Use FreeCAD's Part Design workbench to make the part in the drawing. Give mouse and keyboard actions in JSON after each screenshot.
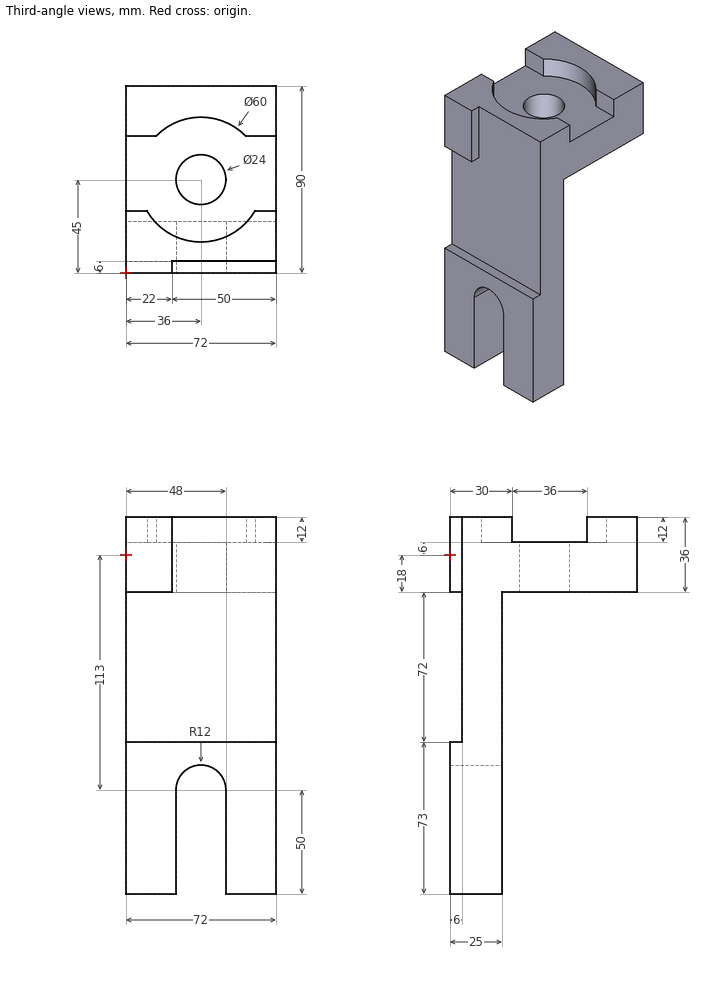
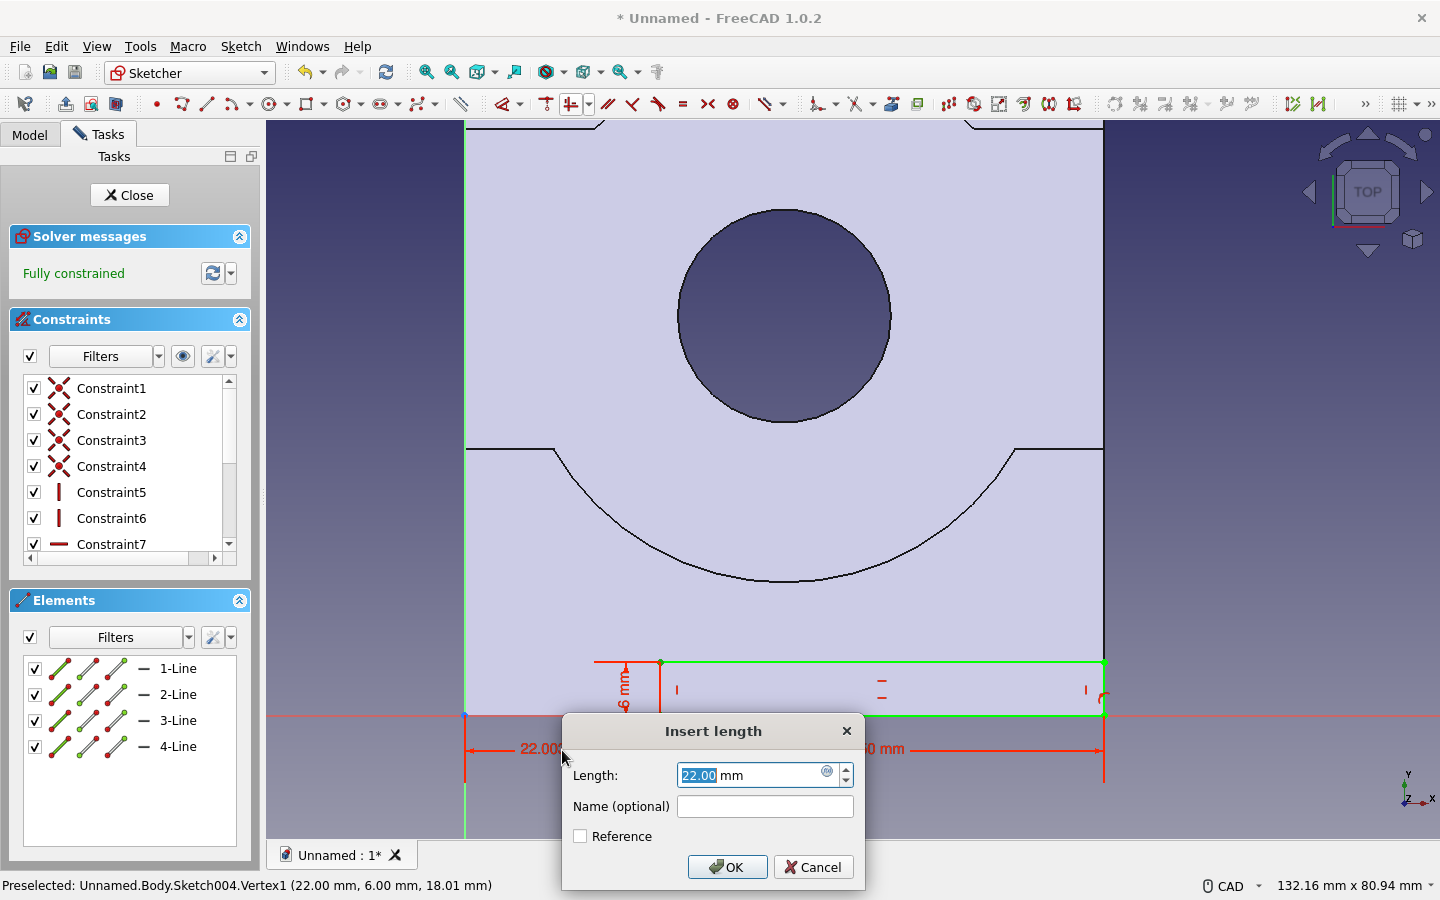
{"action": "type", "text": "22"}
{"action": "key", "text": "Return"}
{"action": "key", "text": "Escape"}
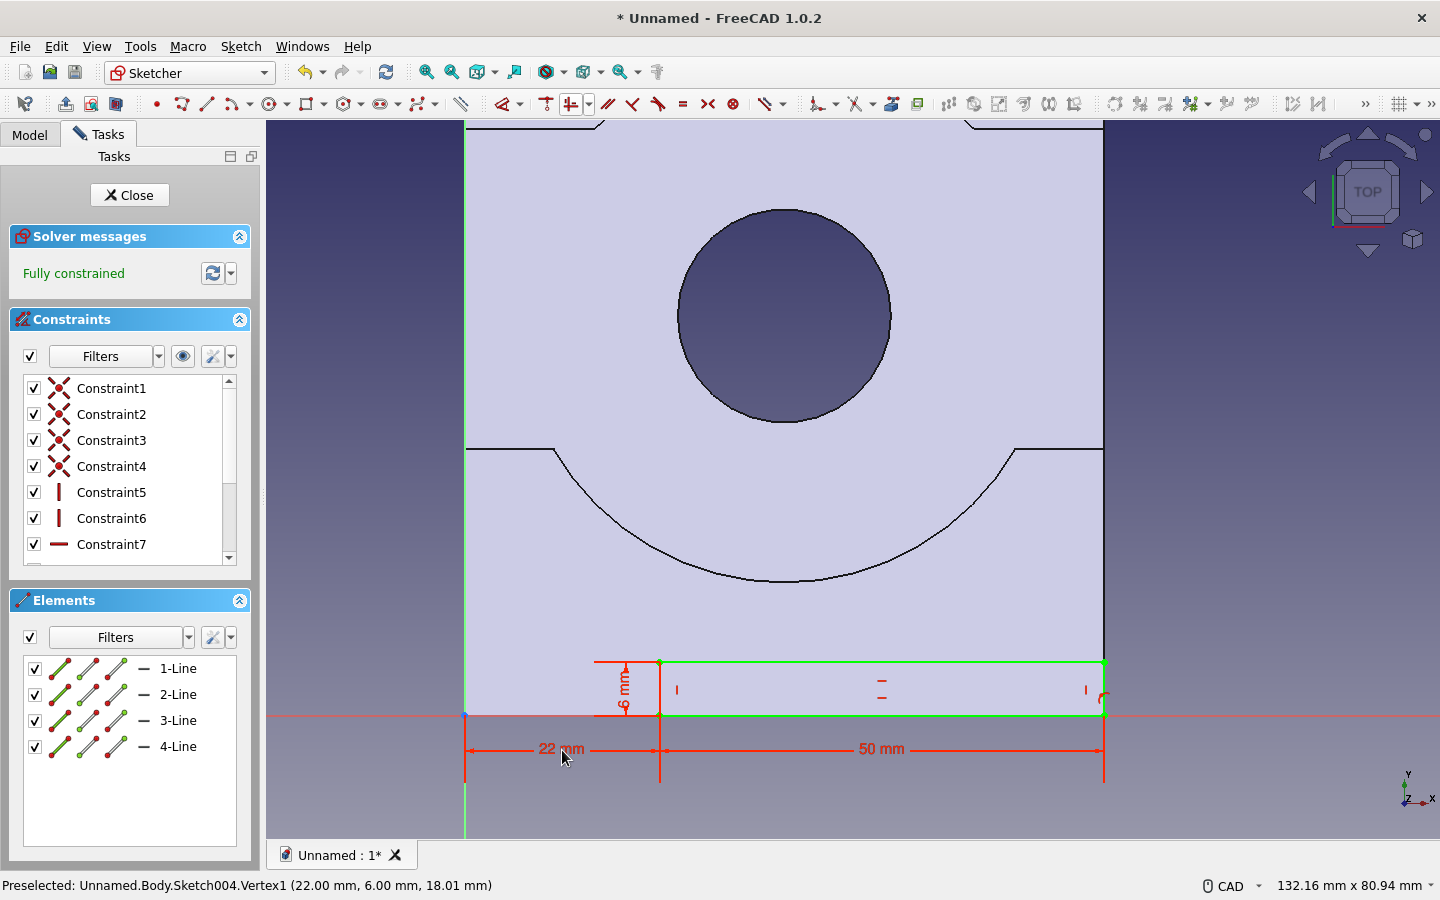
{"action": "left_click", "coordinate": [130, 195]}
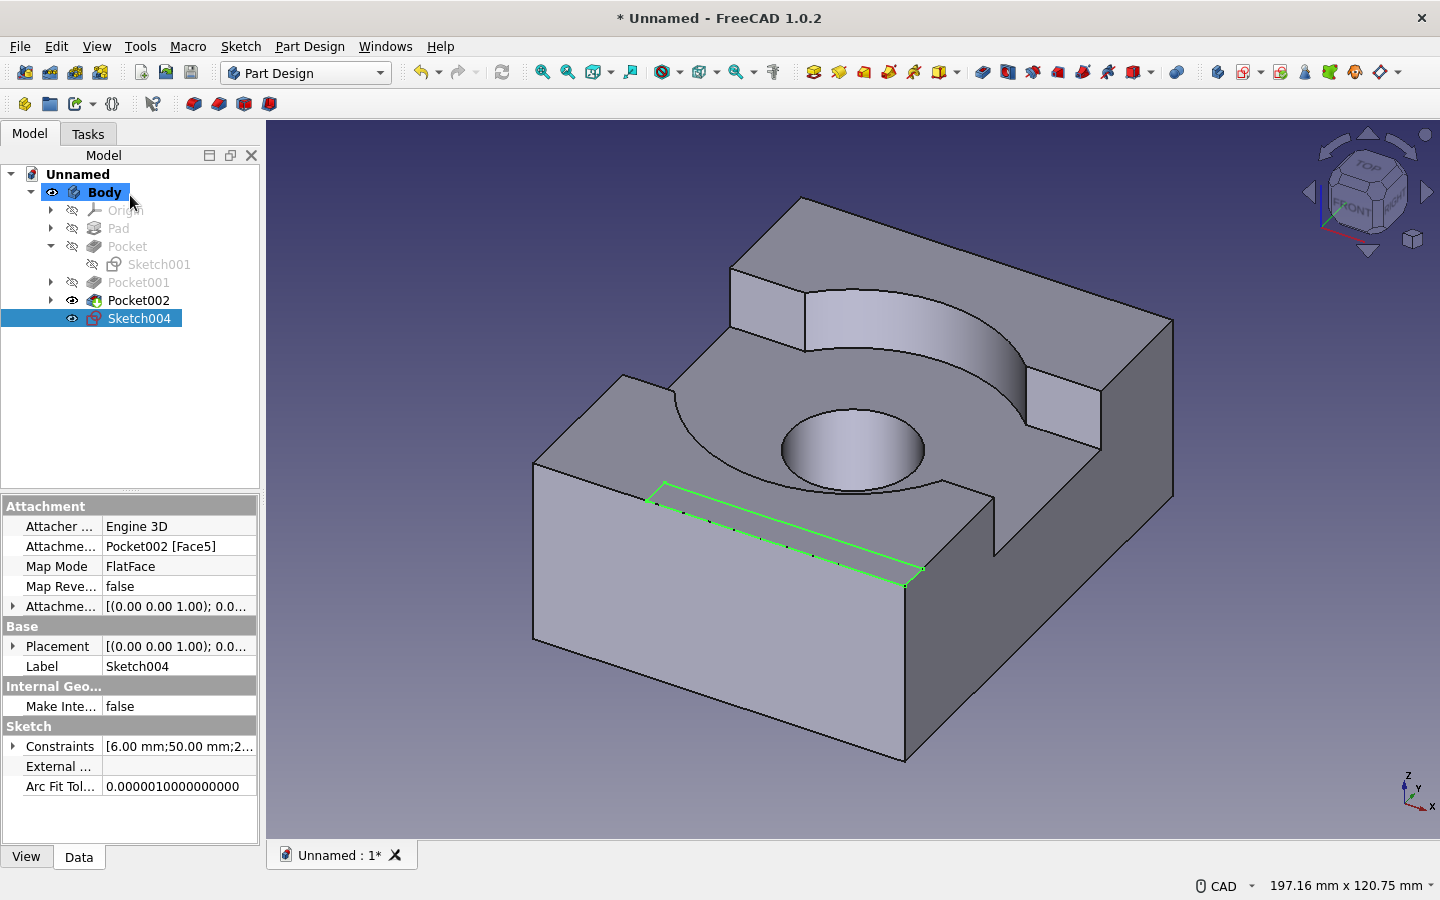
{"action": "left_click", "coordinate": [983, 72]}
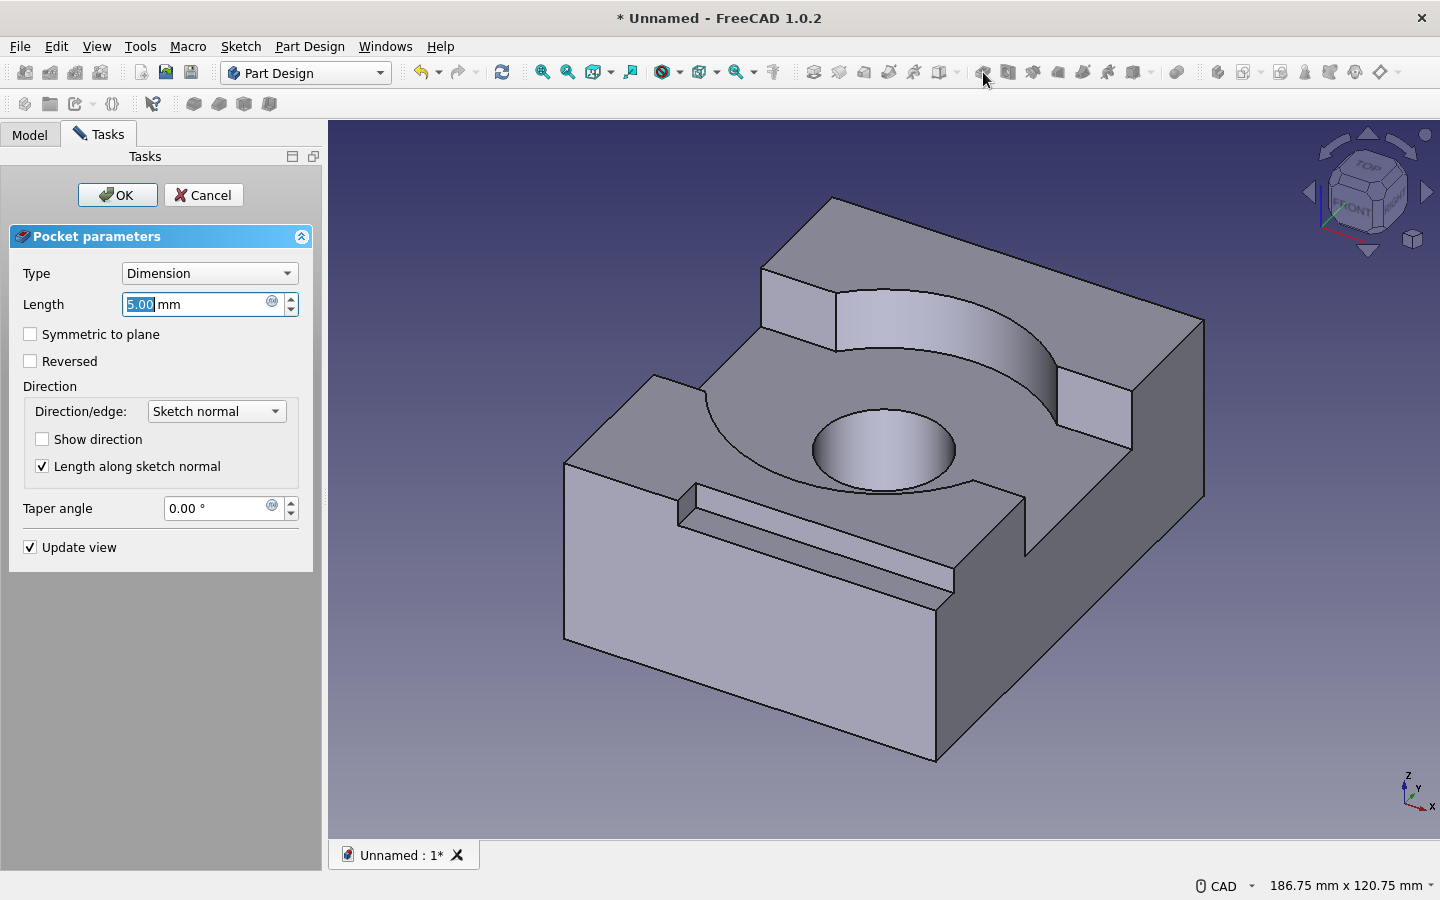
{"action": "left_click", "coordinate": [210, 274]}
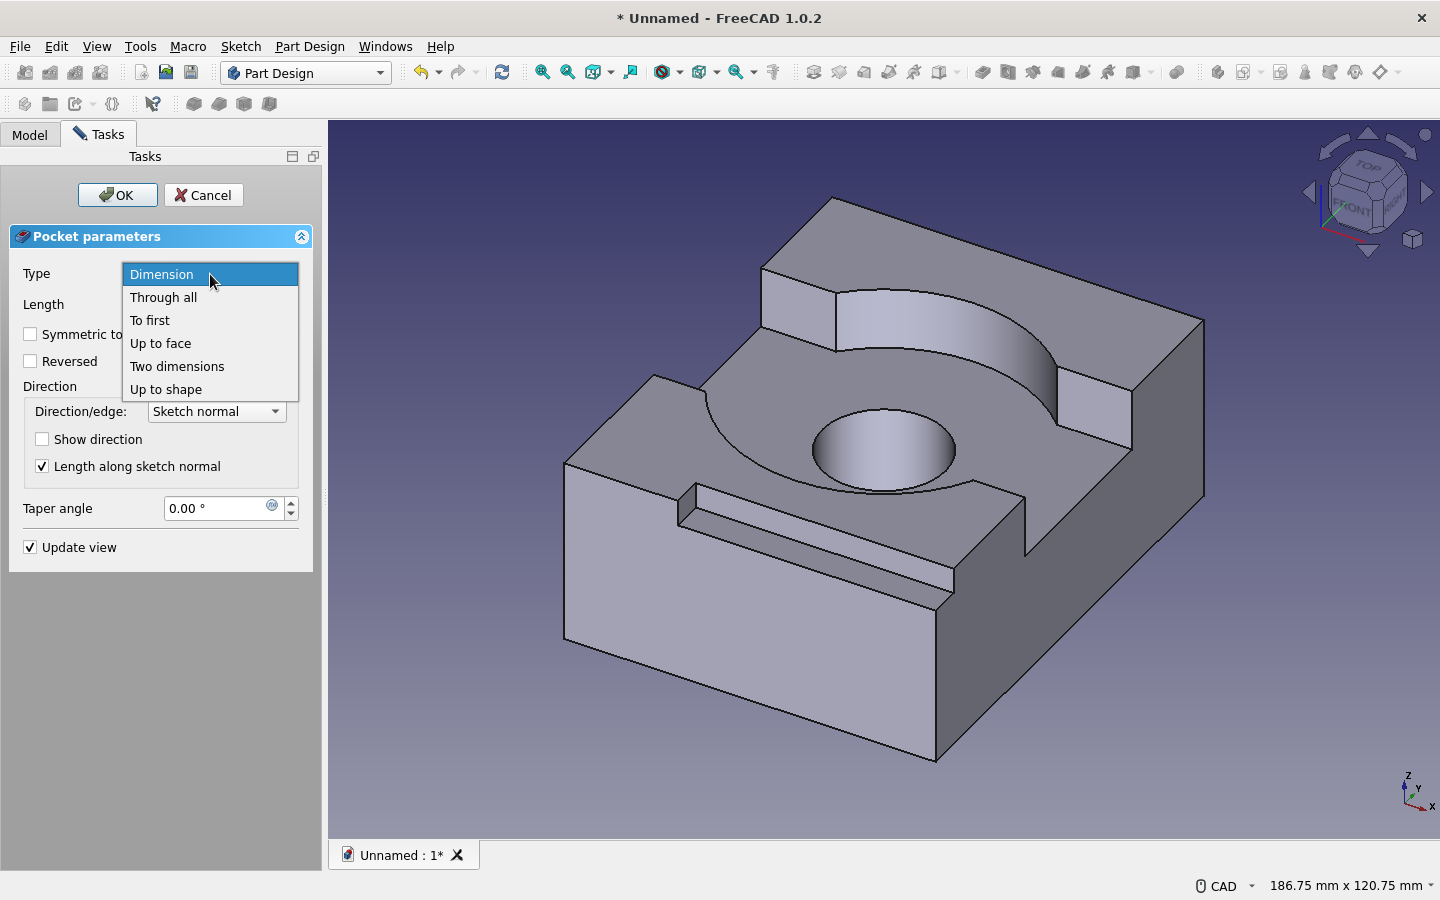
{"action": "left_click", "coordinate": [208, 298]}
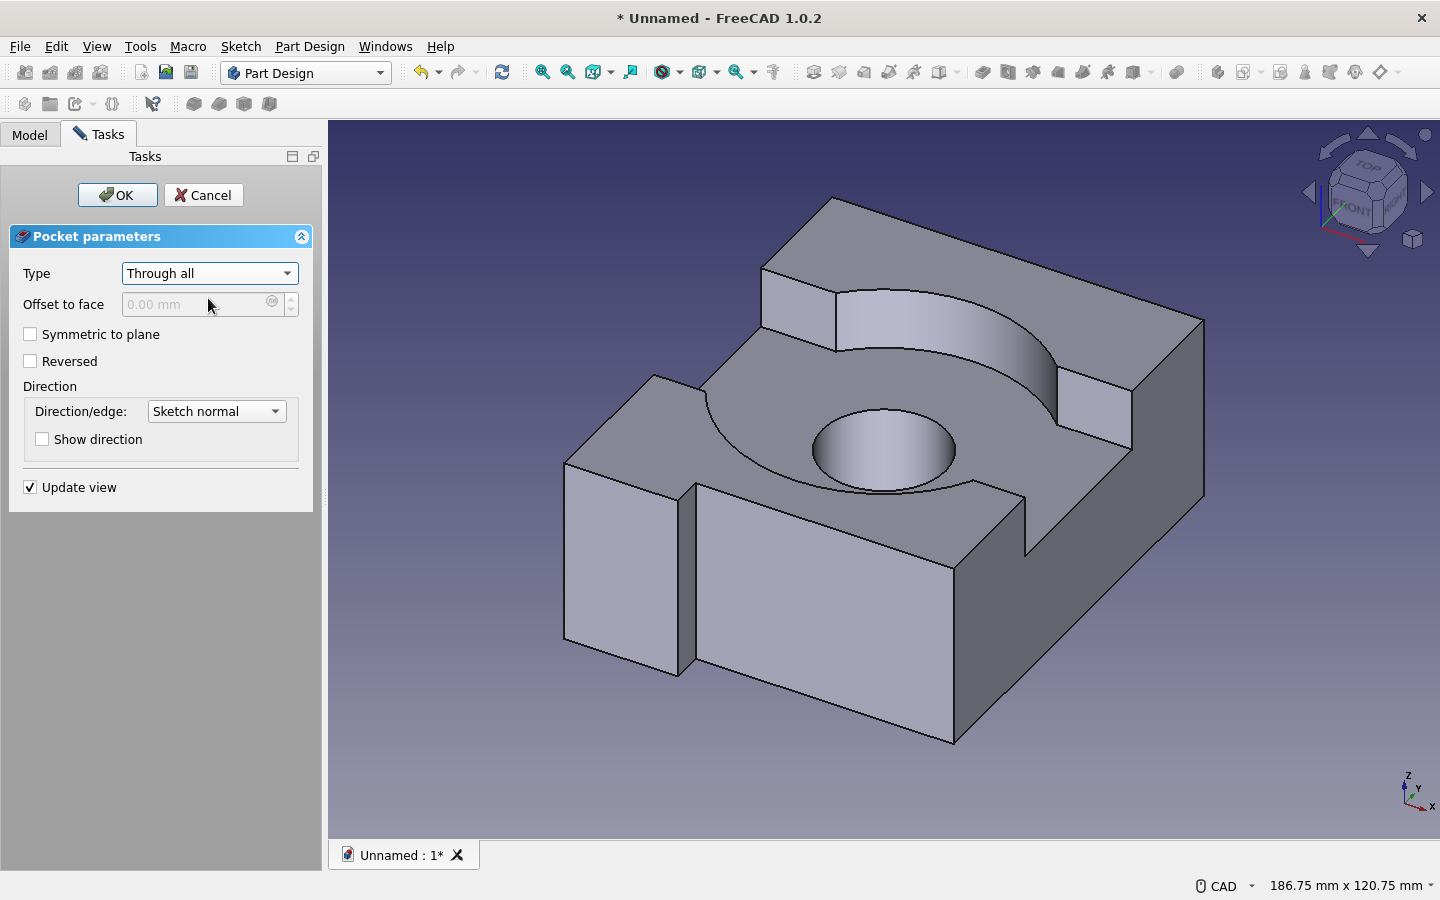
{"action": "left_click", "coordinate": [118, 195]}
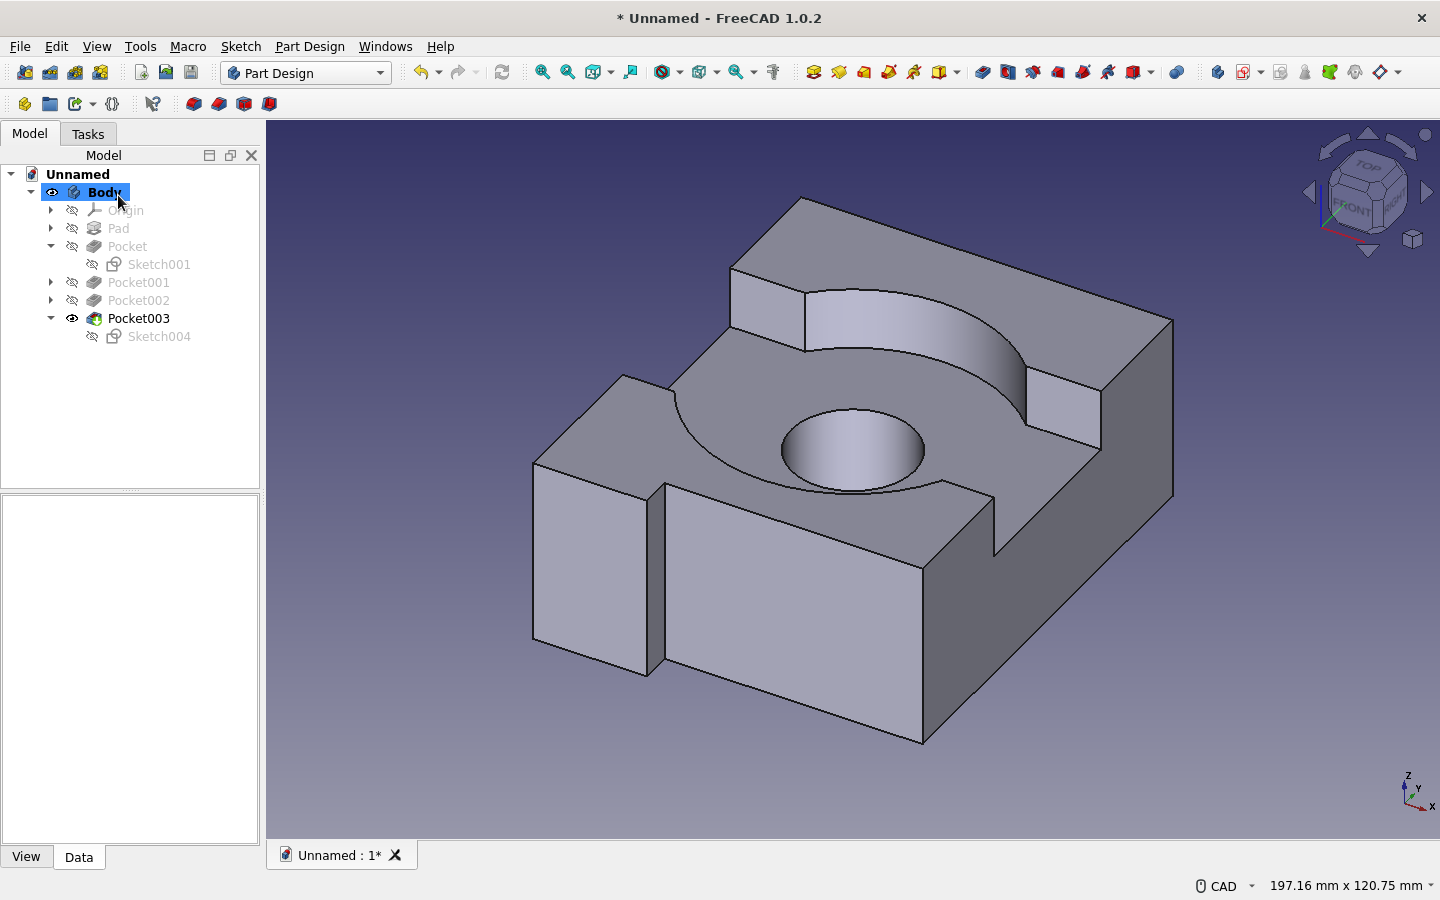
{"action": "left_click", "coordinate": [1119, 485]}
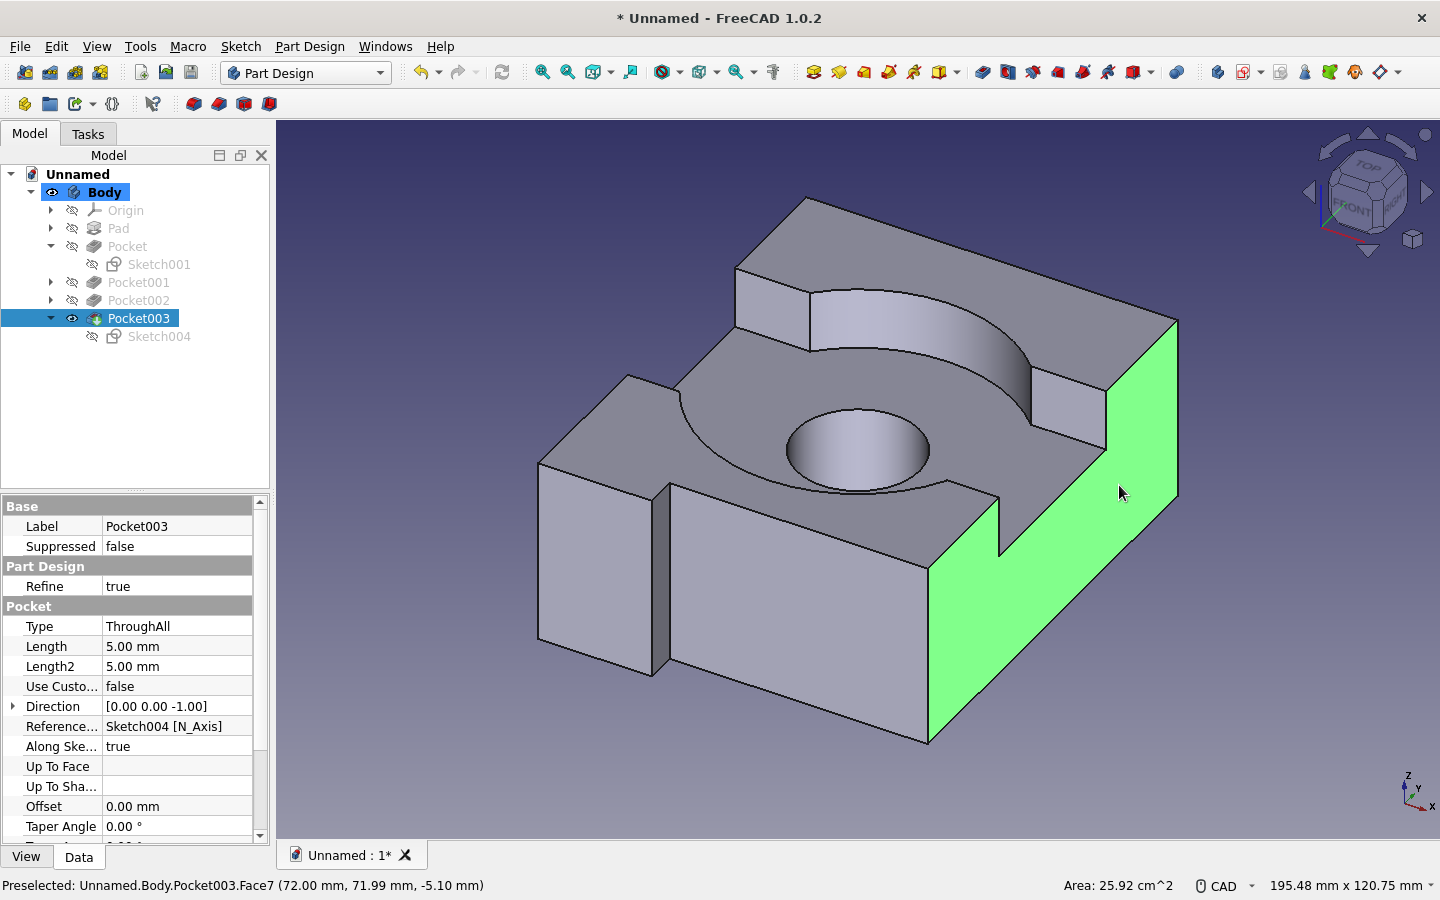
{"action": "left_click", "coordinate": [1242, 72]}